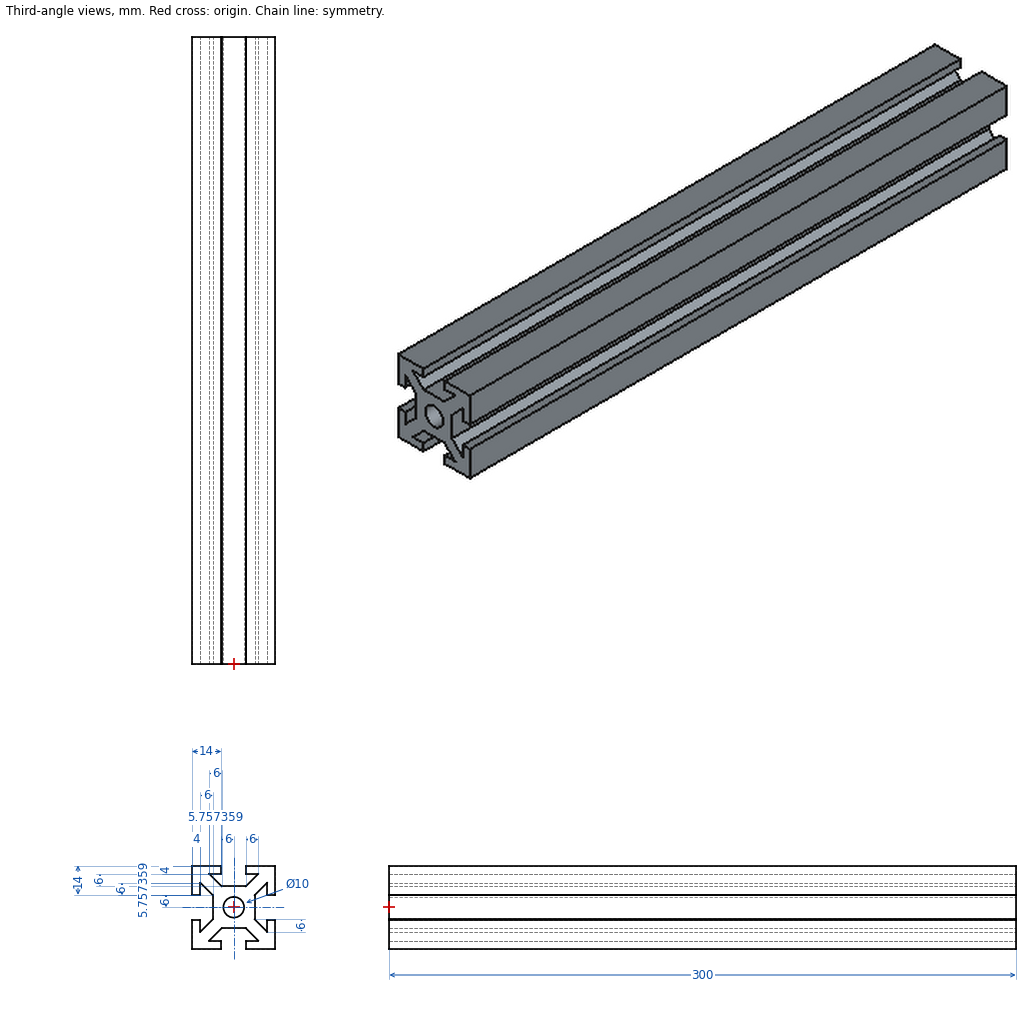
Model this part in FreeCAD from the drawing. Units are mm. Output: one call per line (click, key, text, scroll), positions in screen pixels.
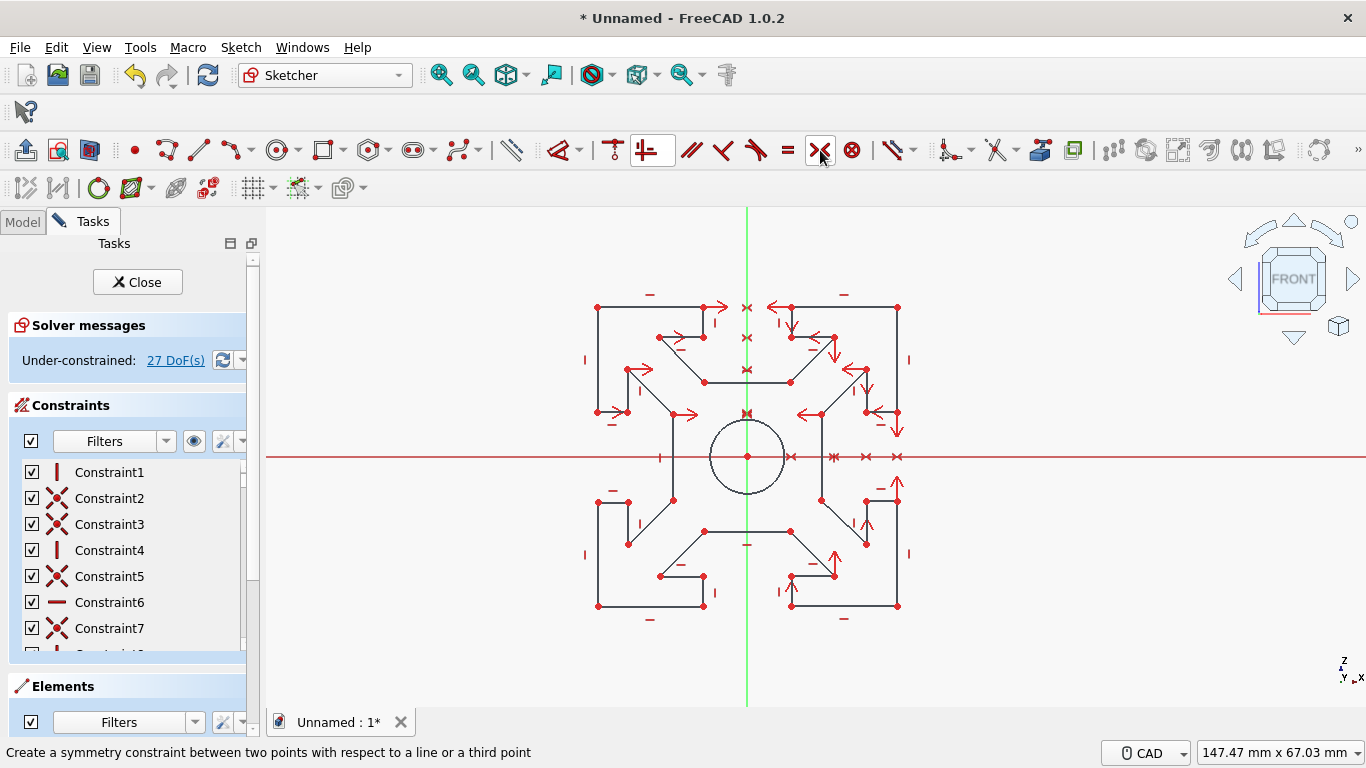
click(790, 383)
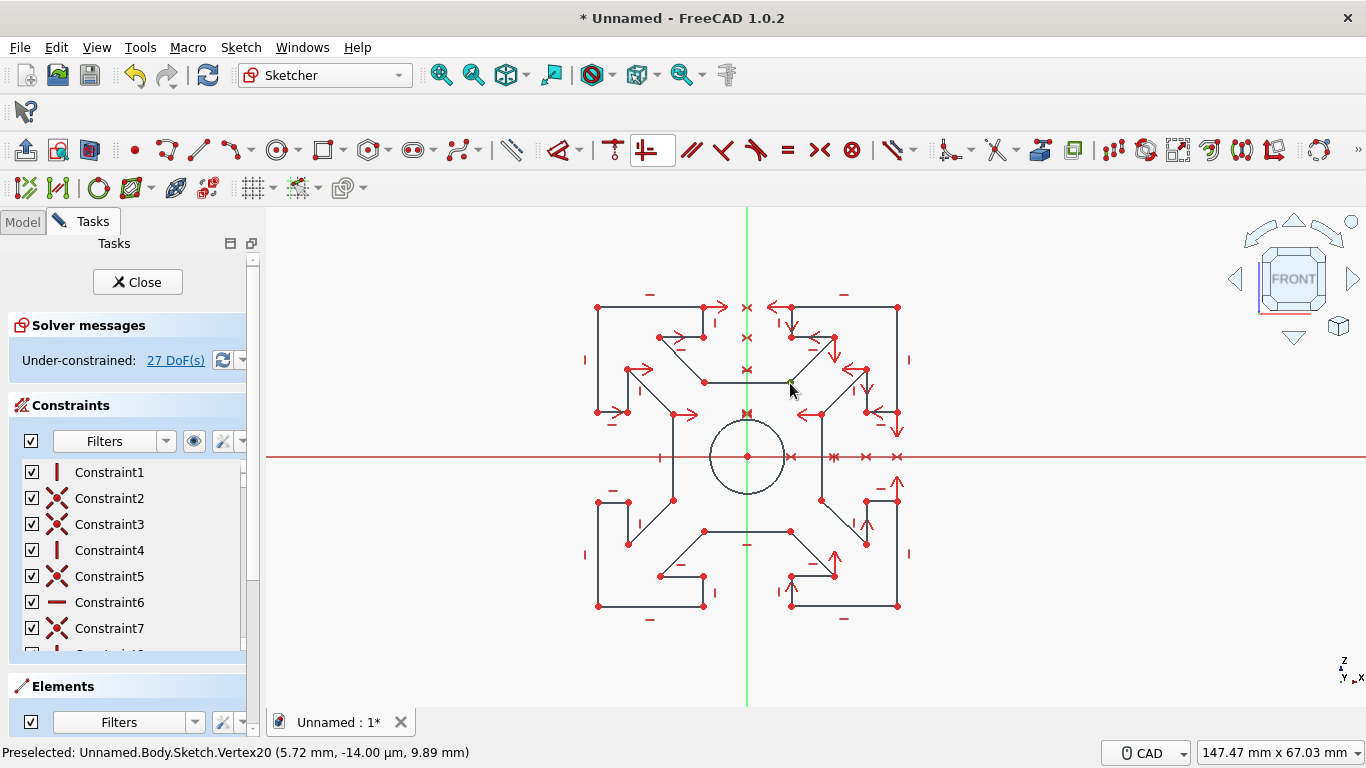
click(790, 532)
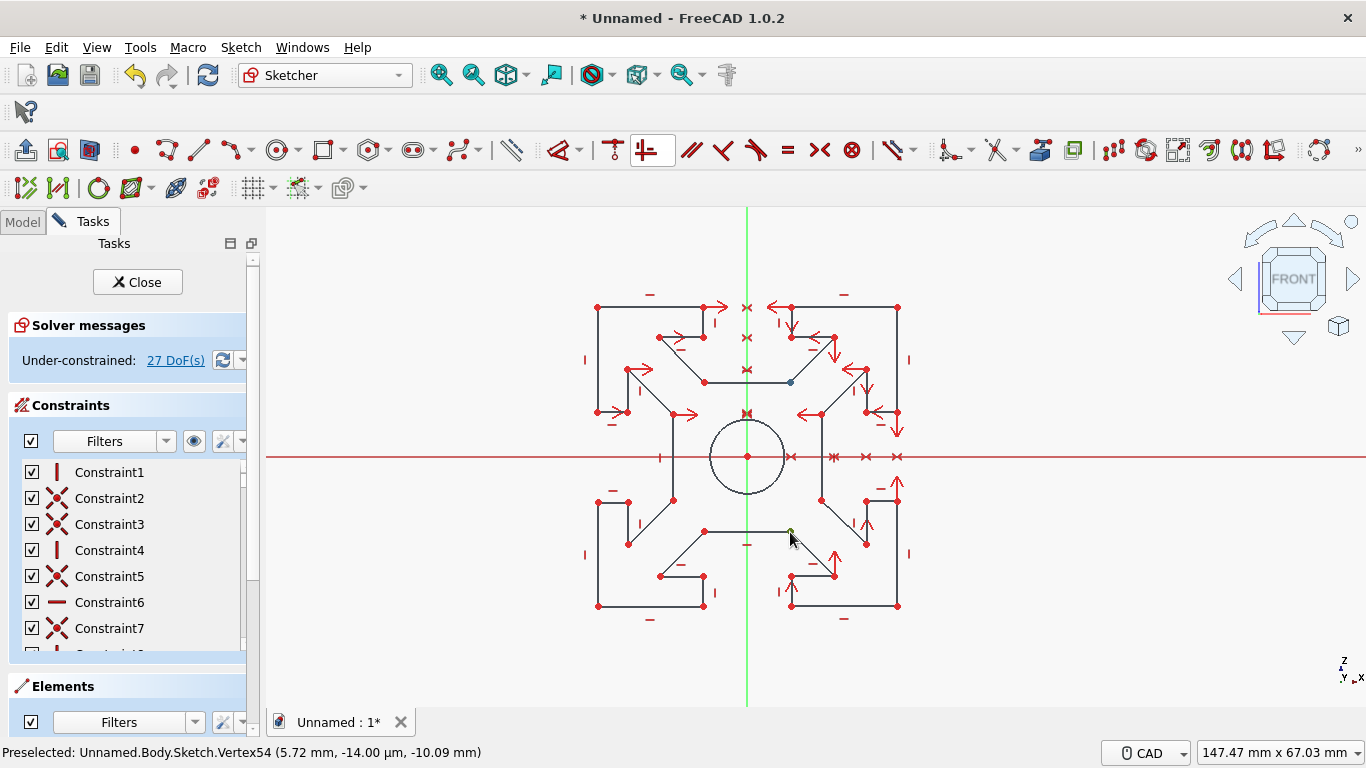
click(359, 457)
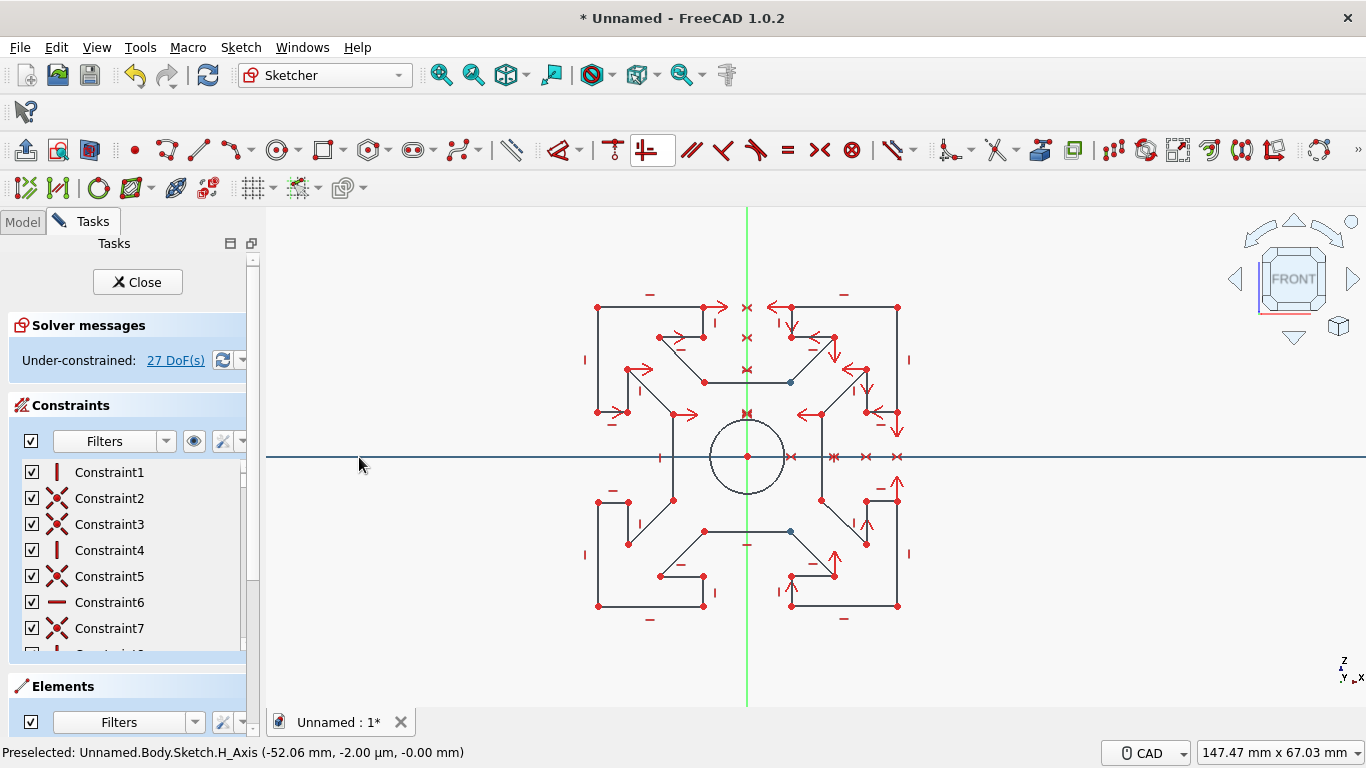
click(820, 150)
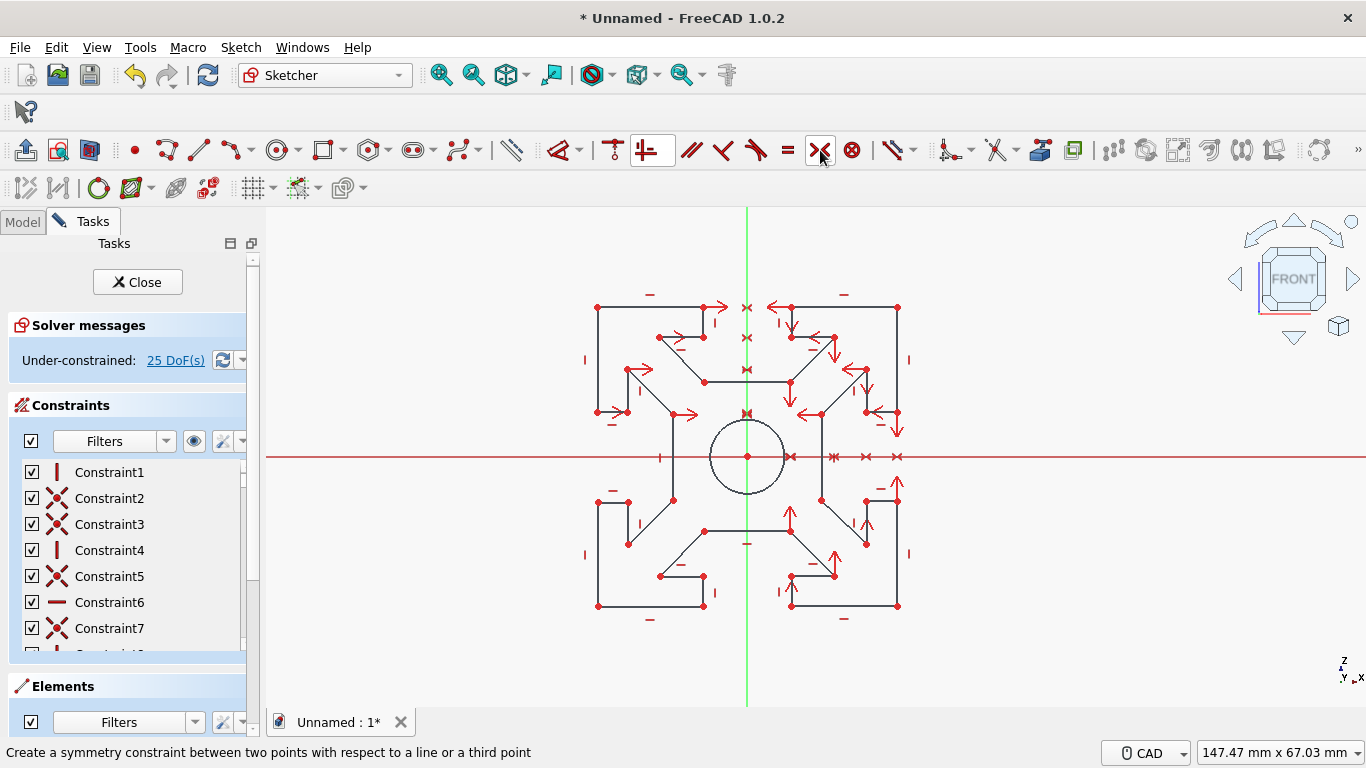
click(660, 337)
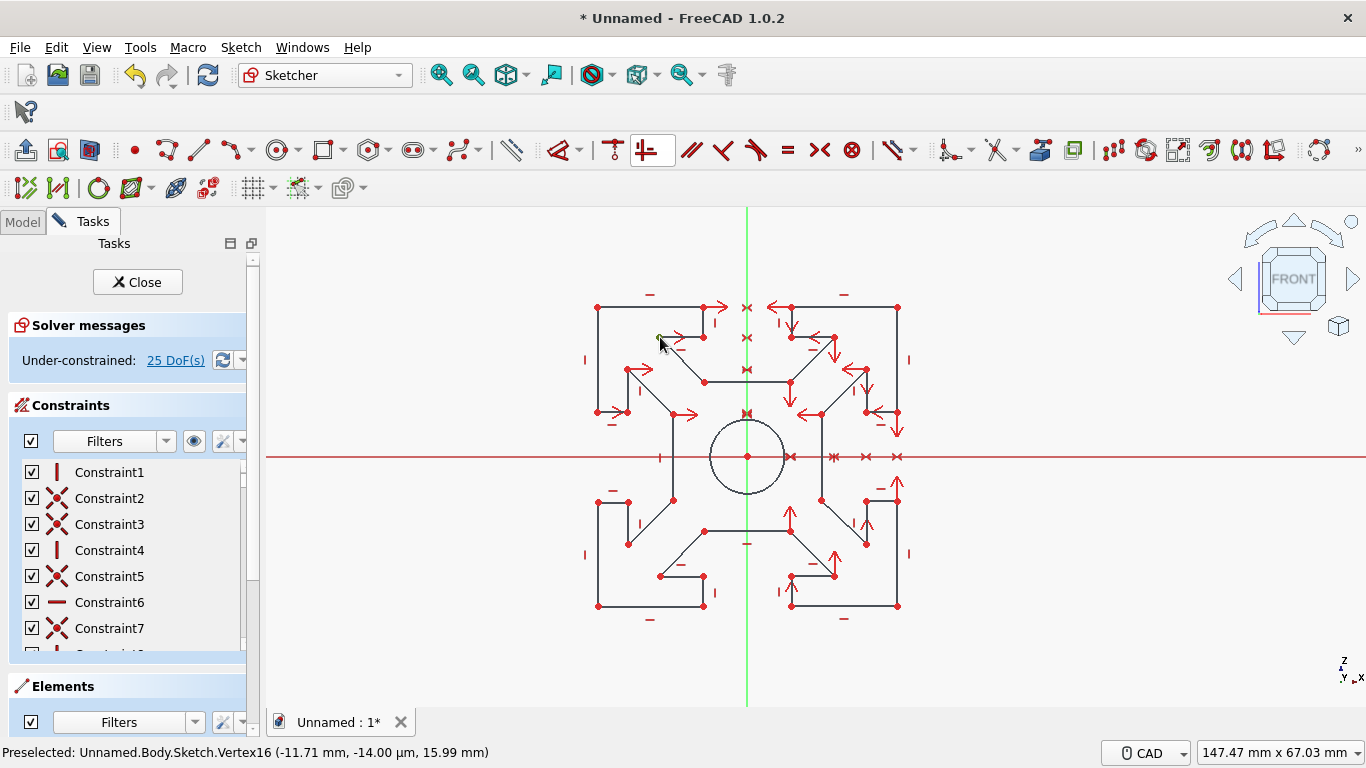
click(660, 577)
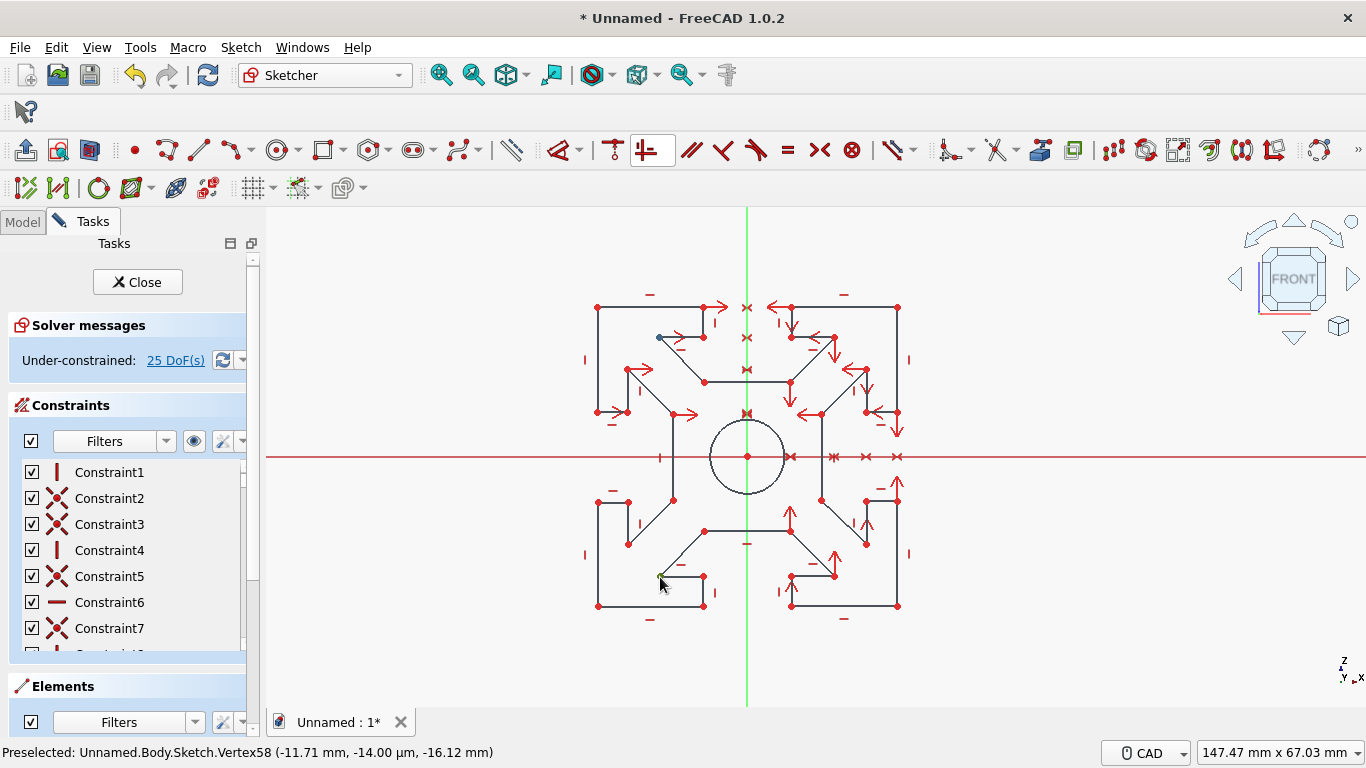
click(359, 457)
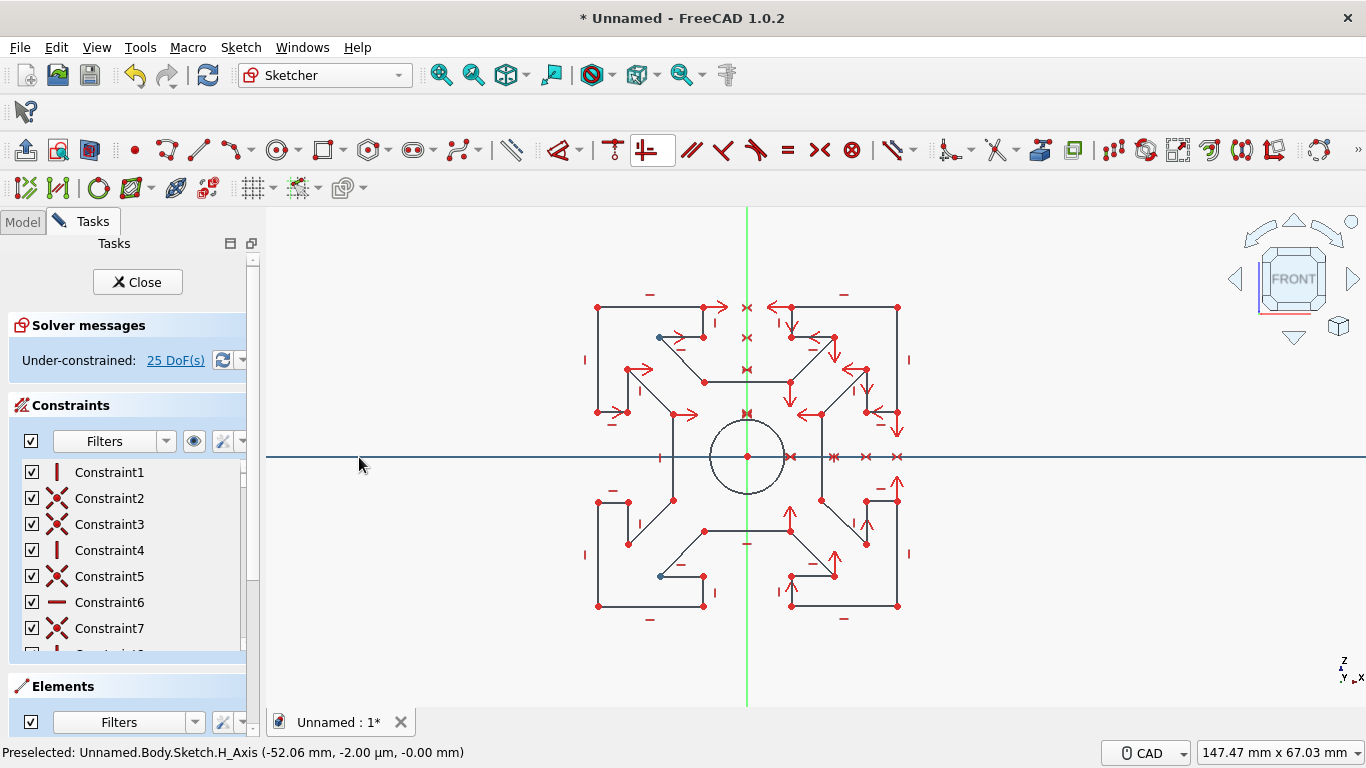
click(820, 150)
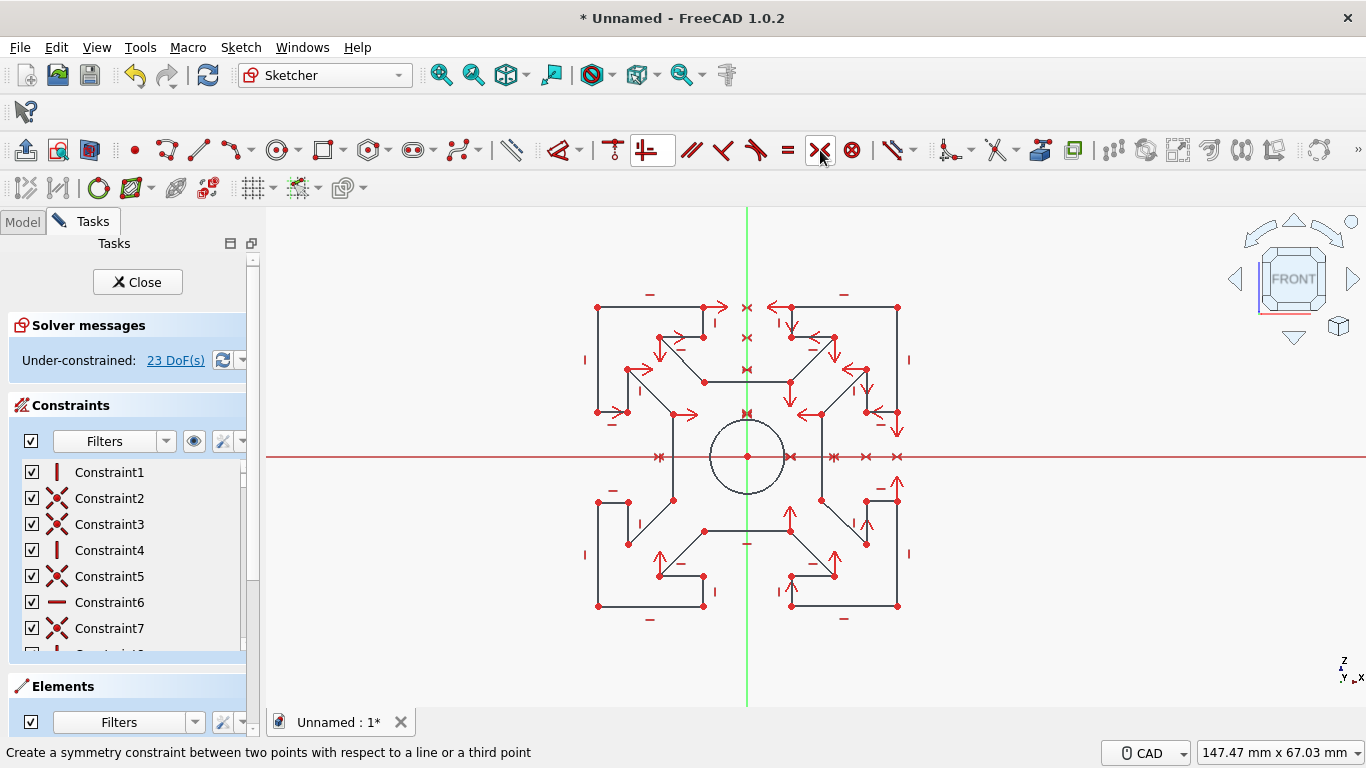
click(703, 307)